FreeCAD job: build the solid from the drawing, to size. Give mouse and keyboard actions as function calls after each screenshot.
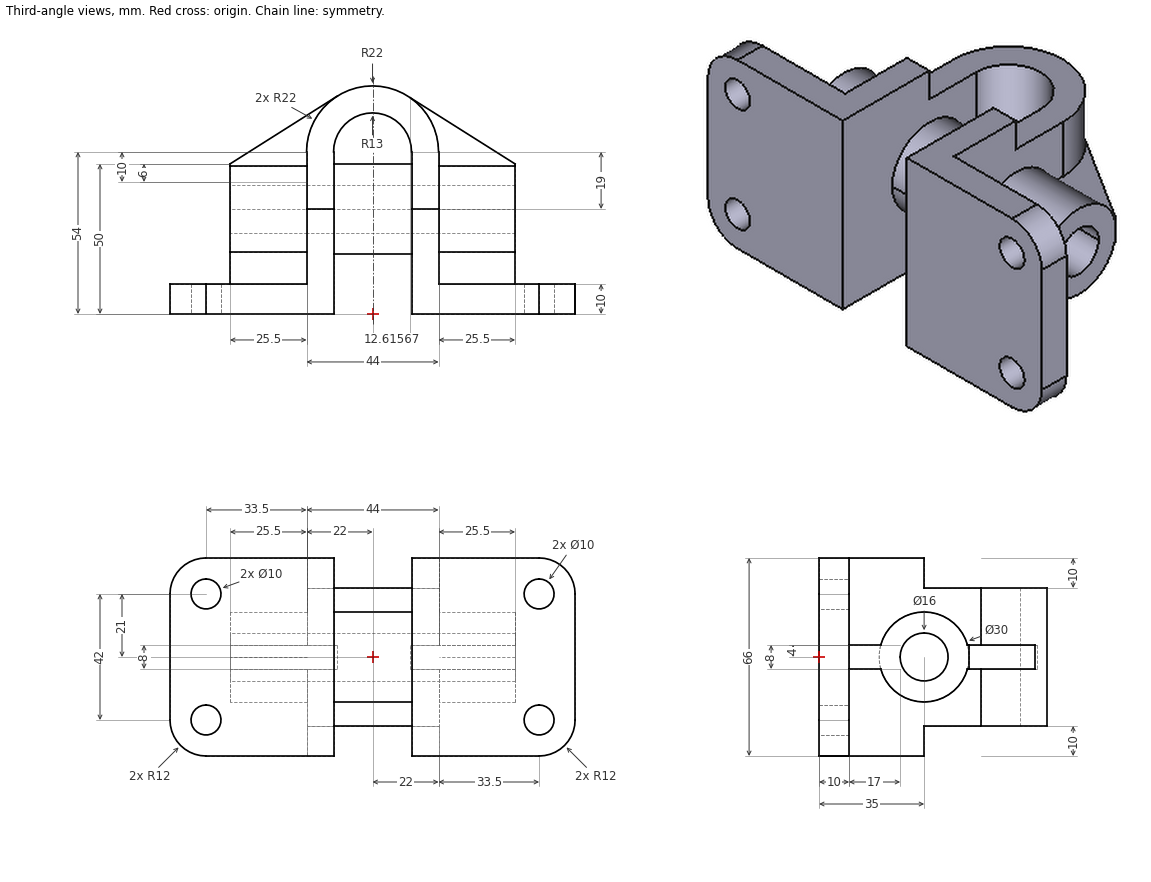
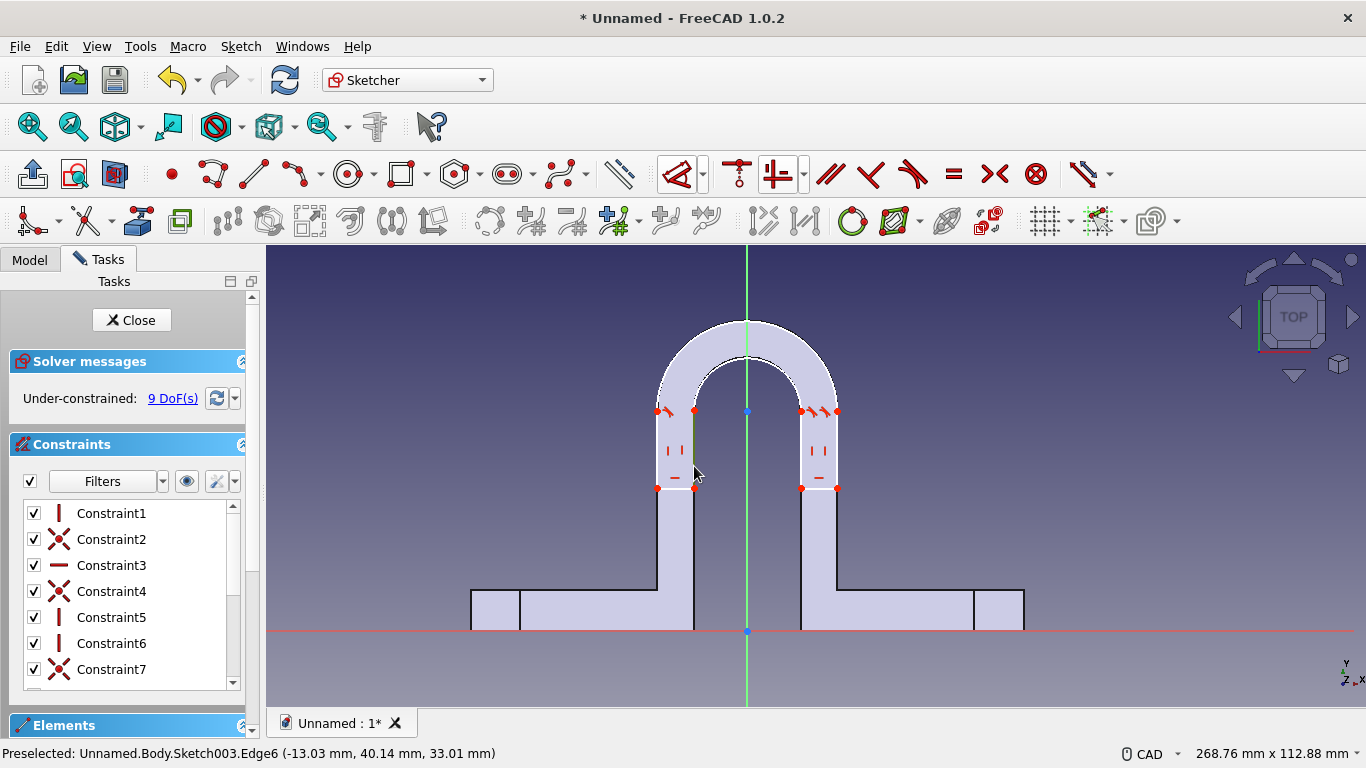
click(779, 369)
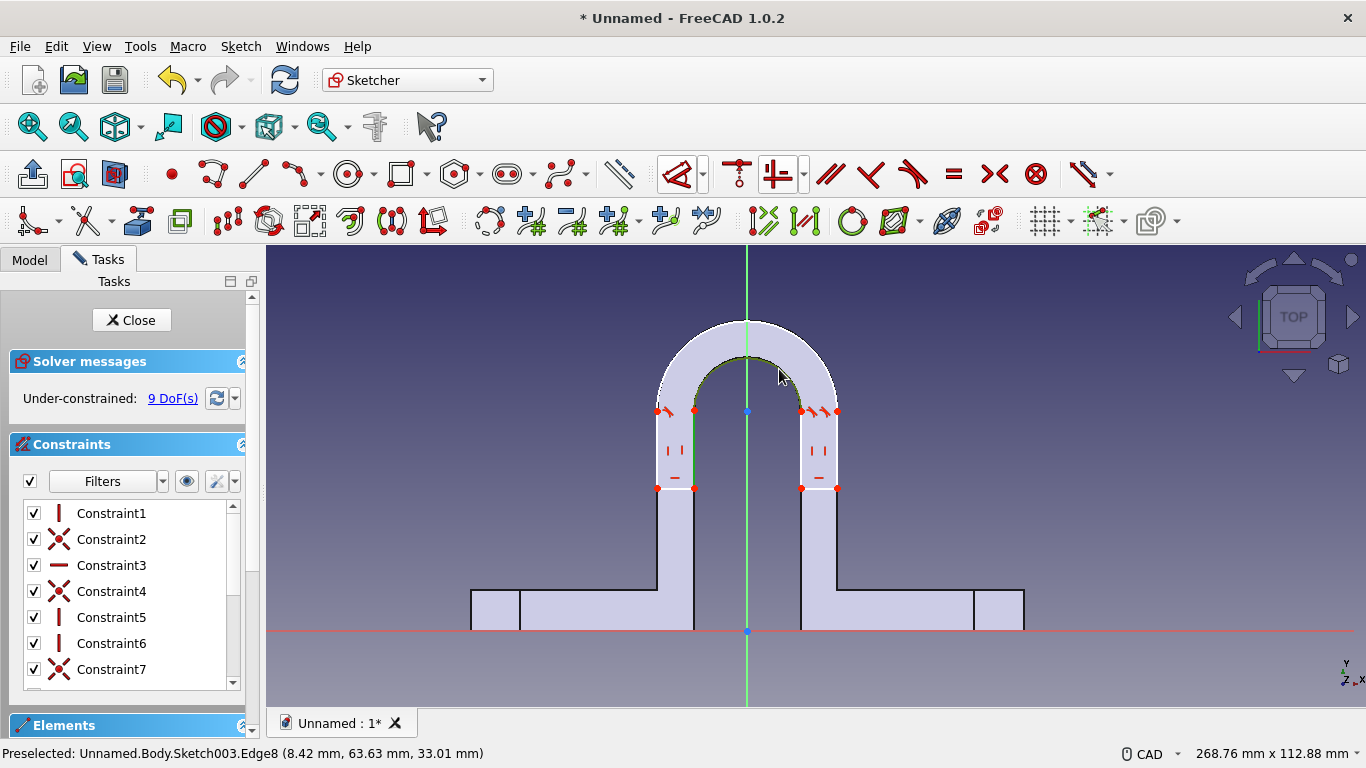
click(913, 174)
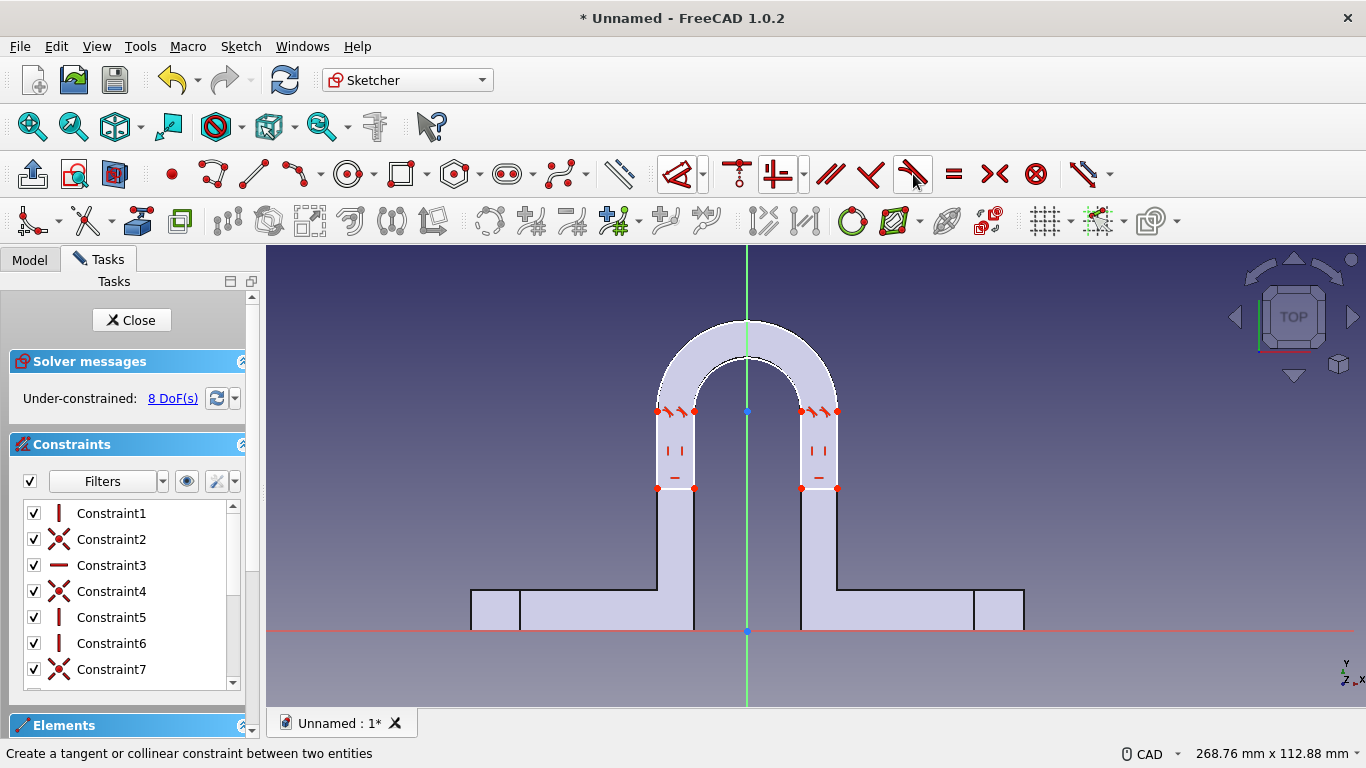
click(800, 339)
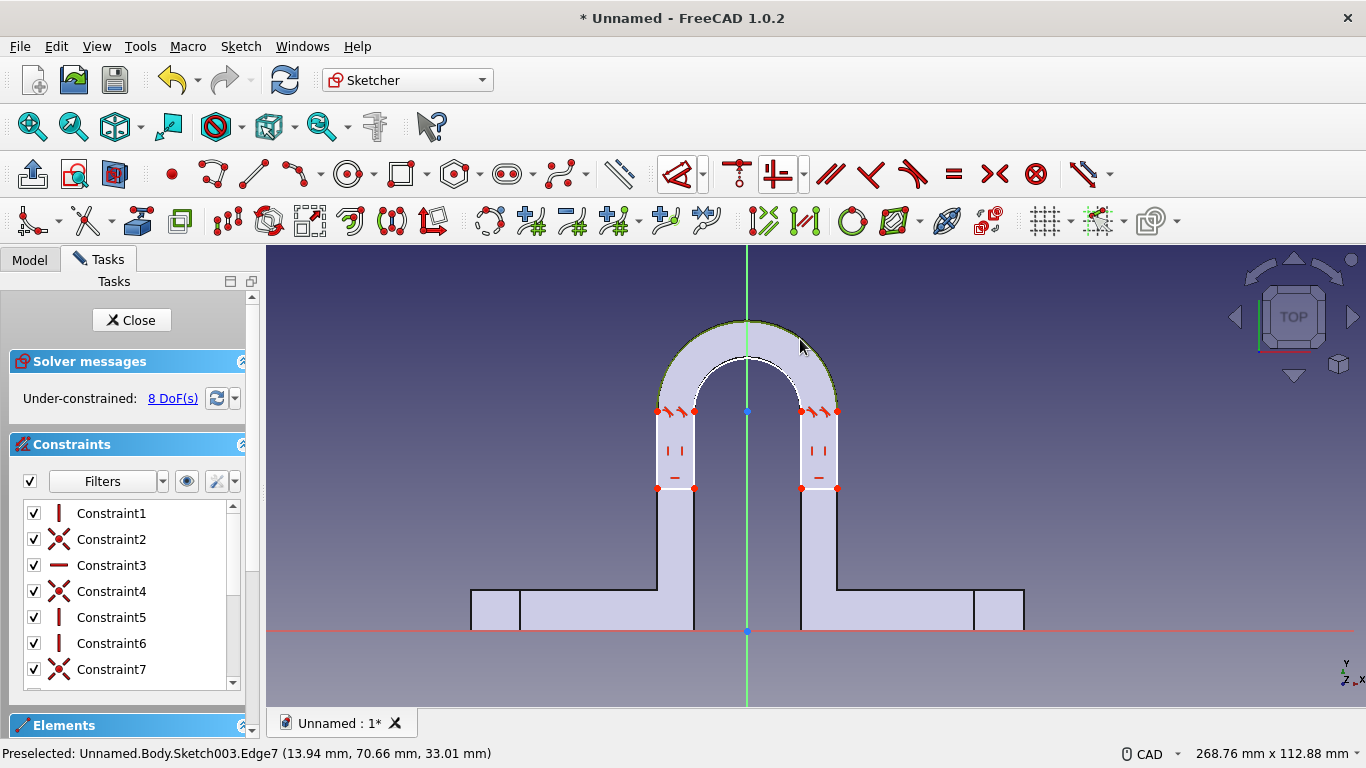
click(779, 369)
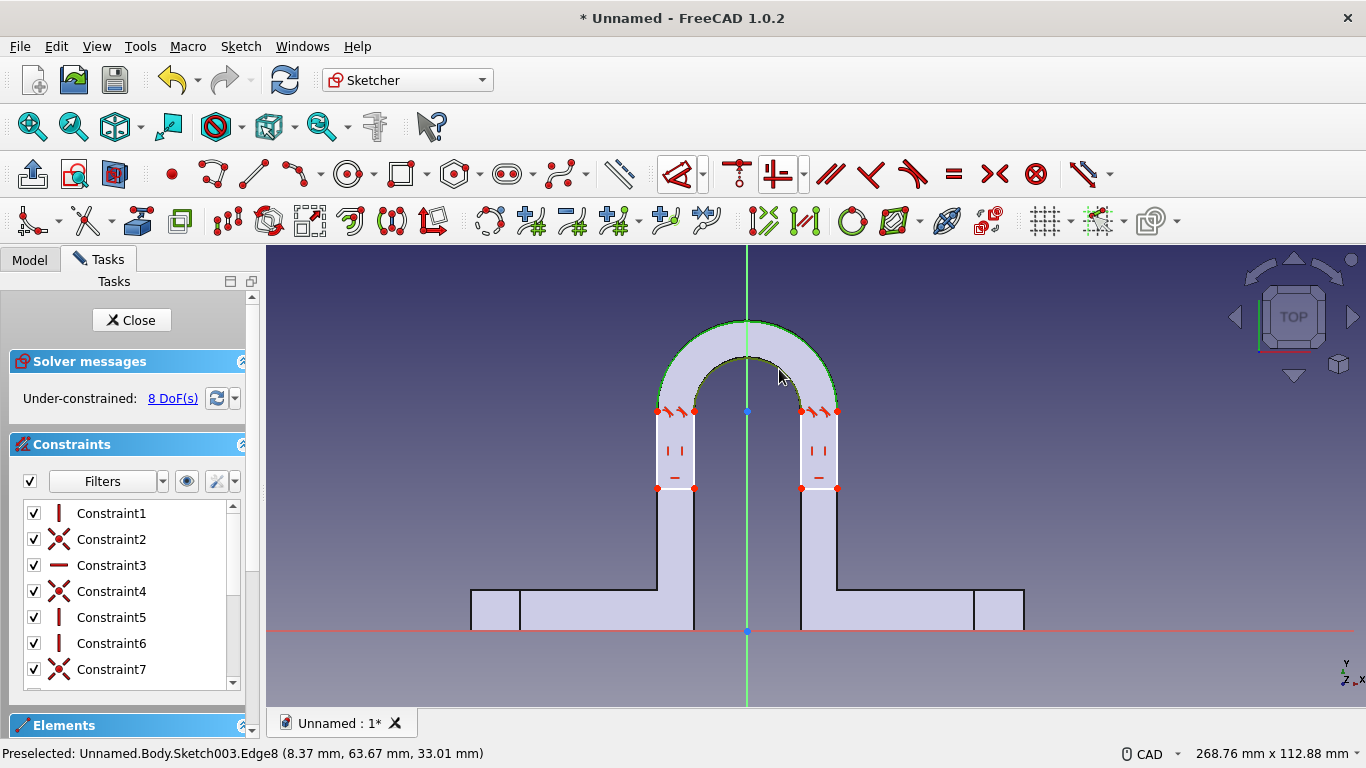
click(737, 174)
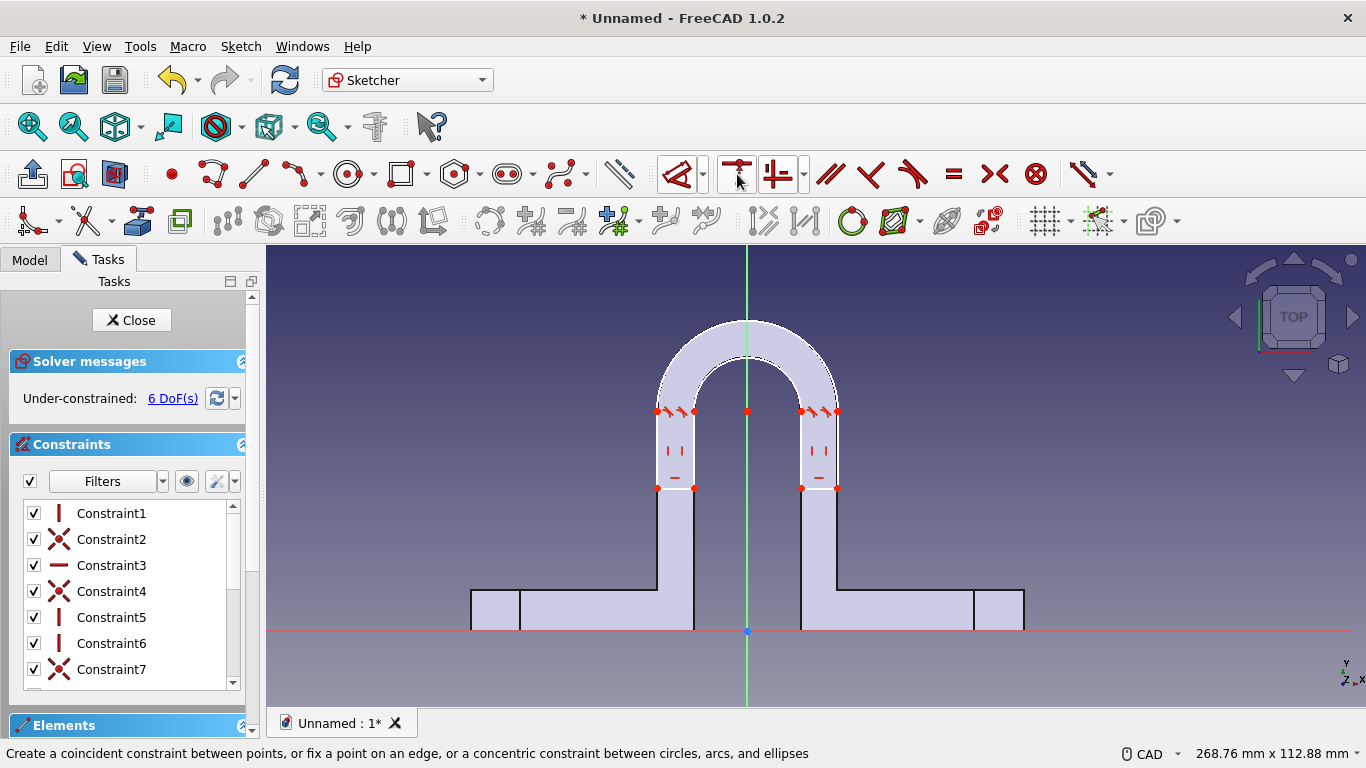
click(748, 411)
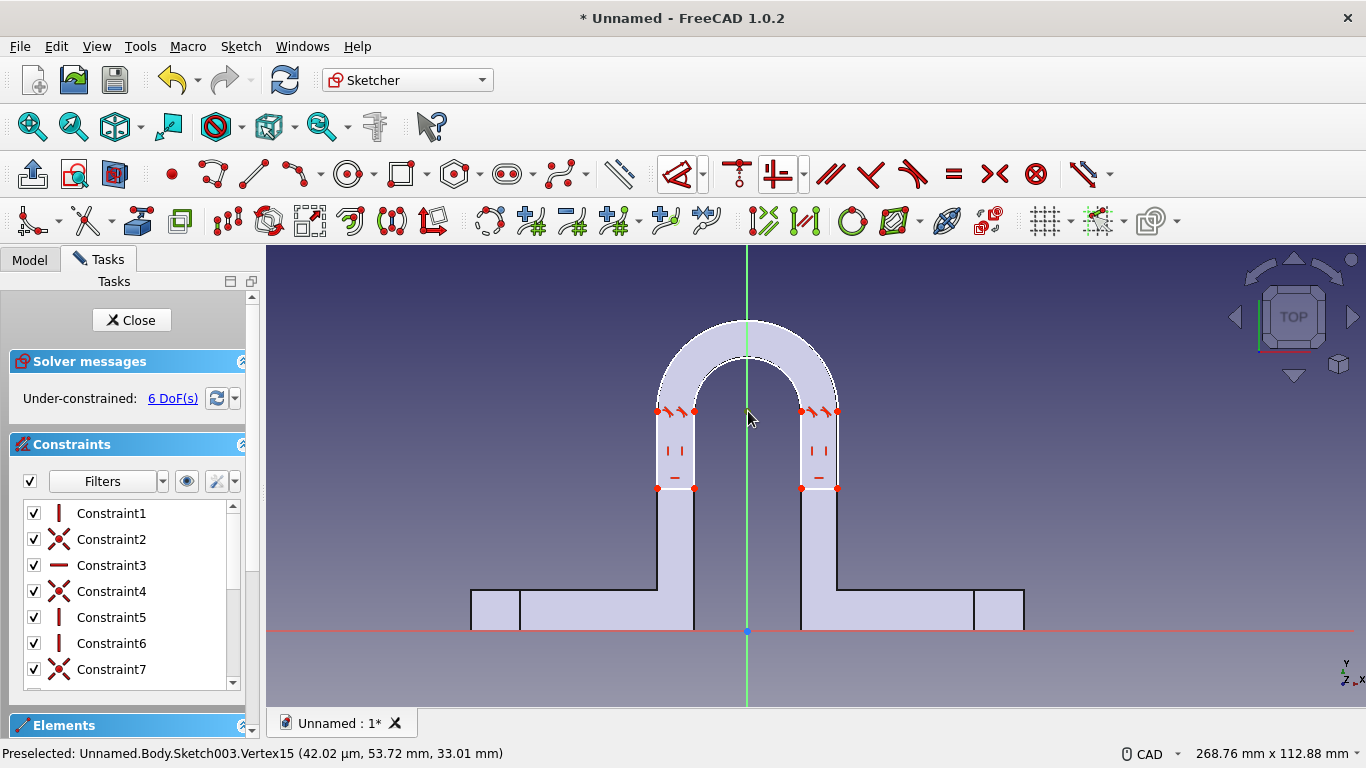
click(747, 592)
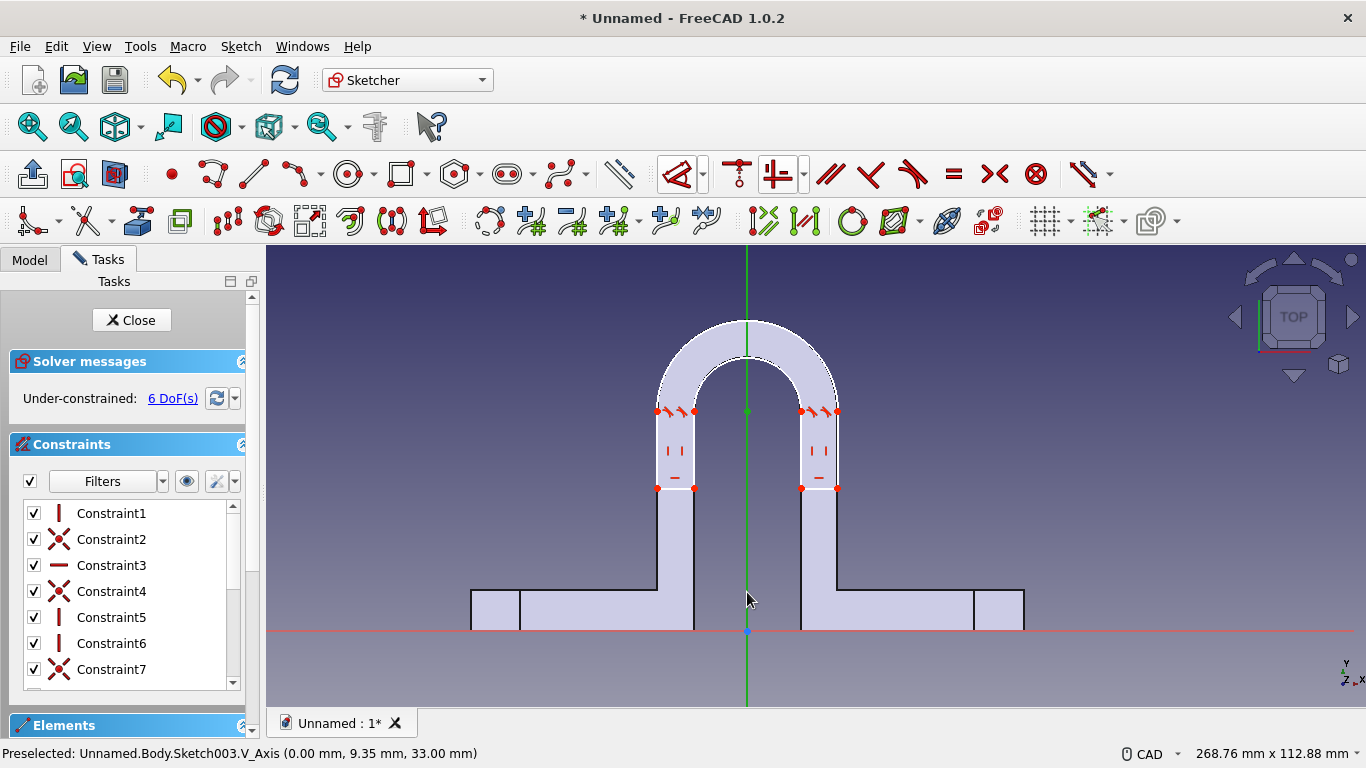
click(737, 174)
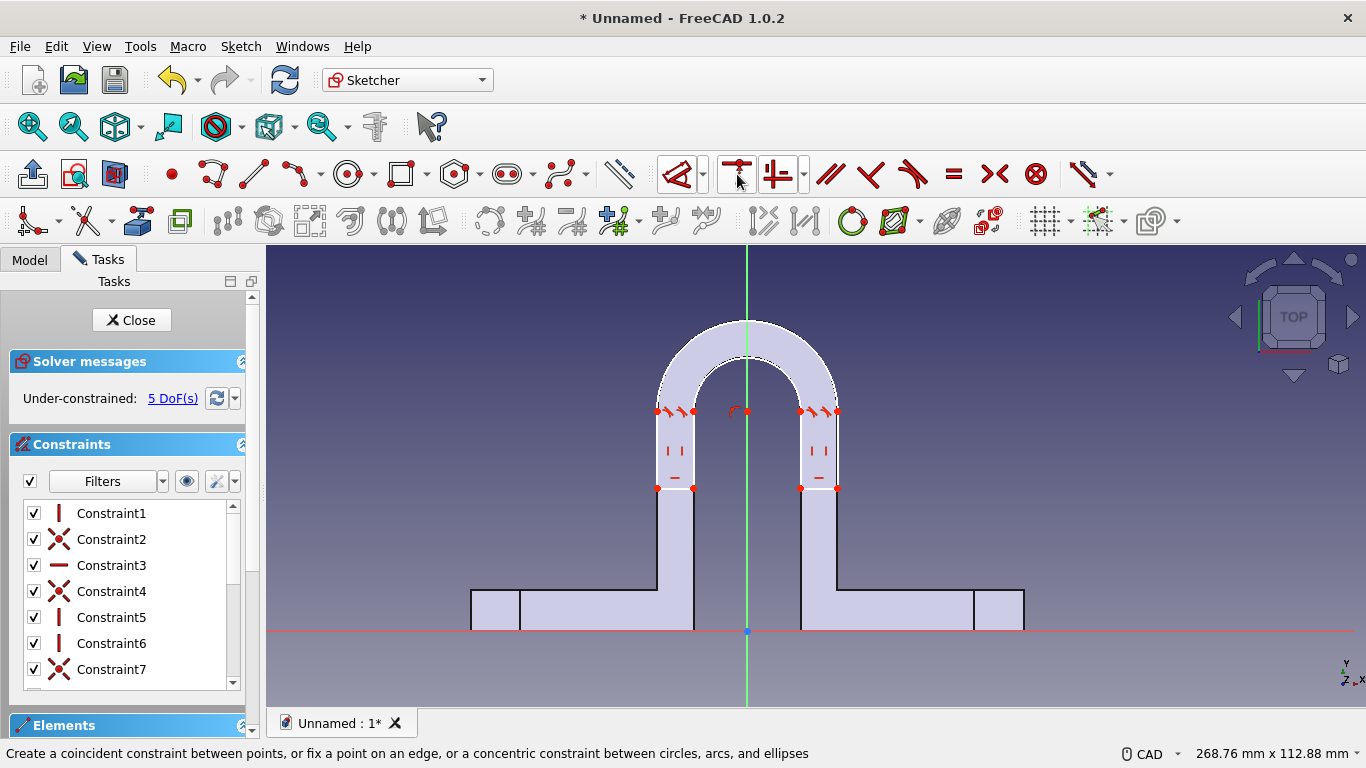
click(800, 338)